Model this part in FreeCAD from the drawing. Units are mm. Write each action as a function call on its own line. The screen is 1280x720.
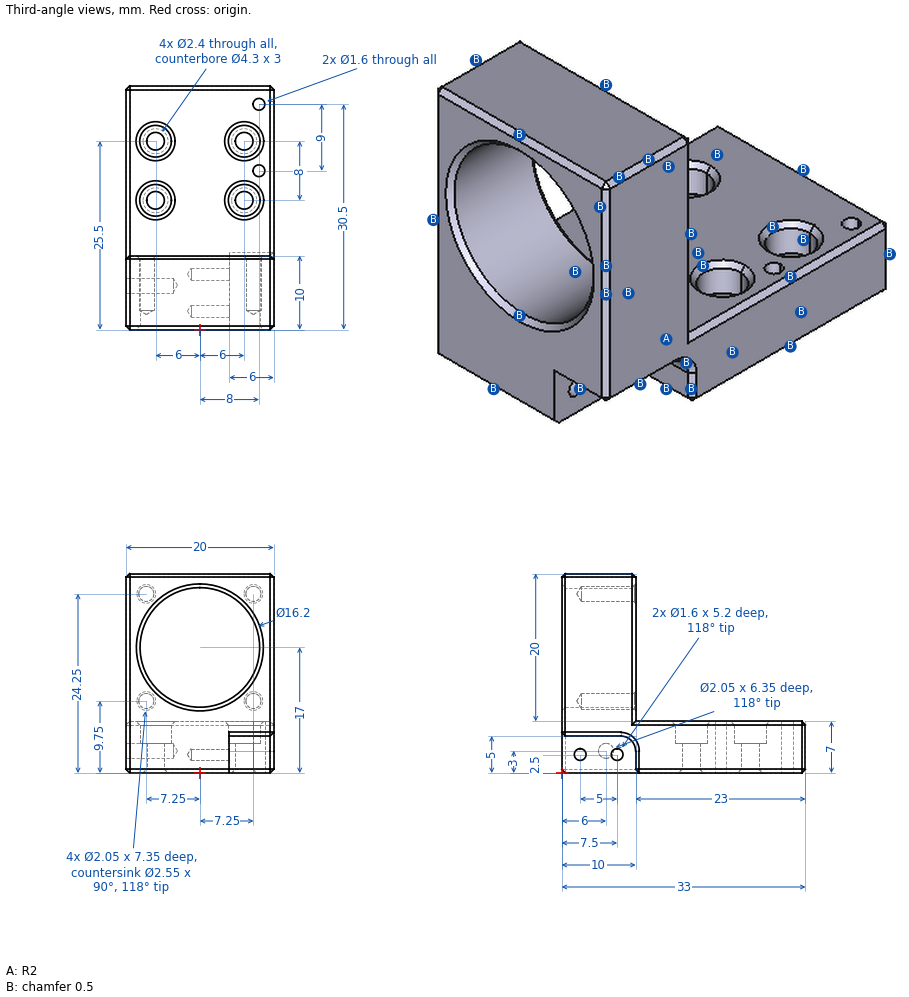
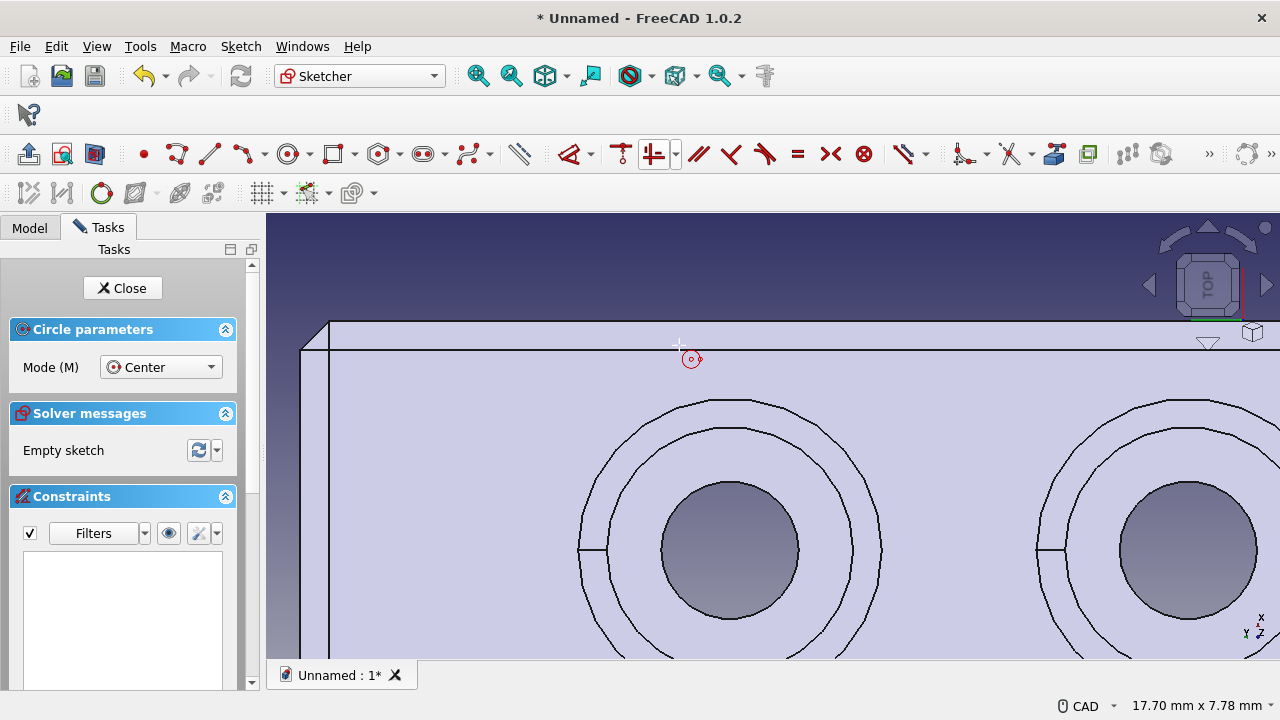
click(444, 436)
move(476, 403)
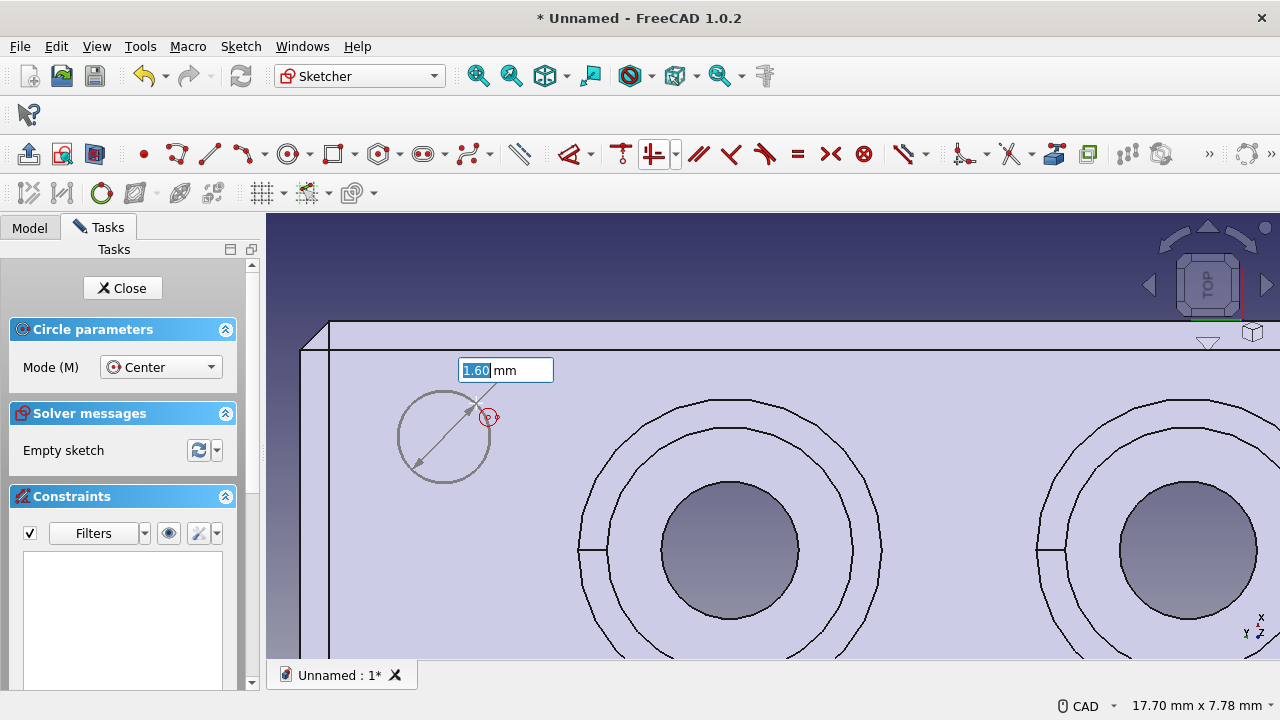
text(1.6)
key(Return)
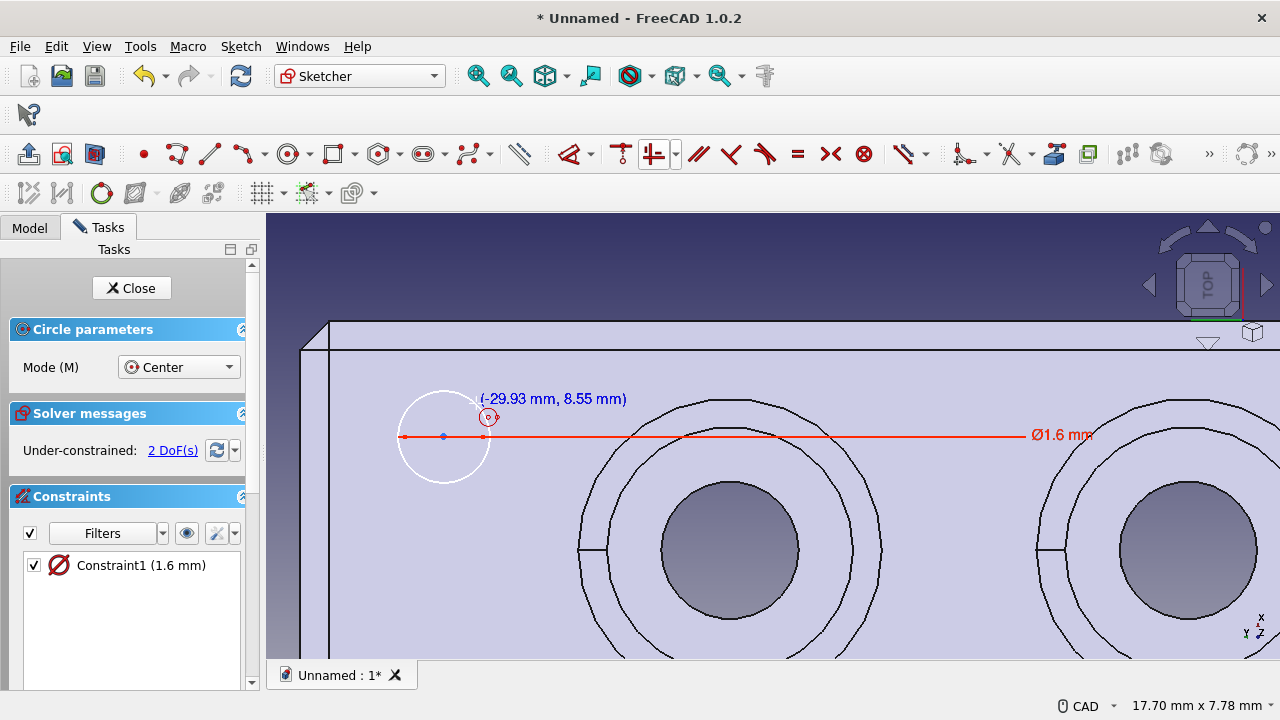
click(959, 436)
move(992, 403)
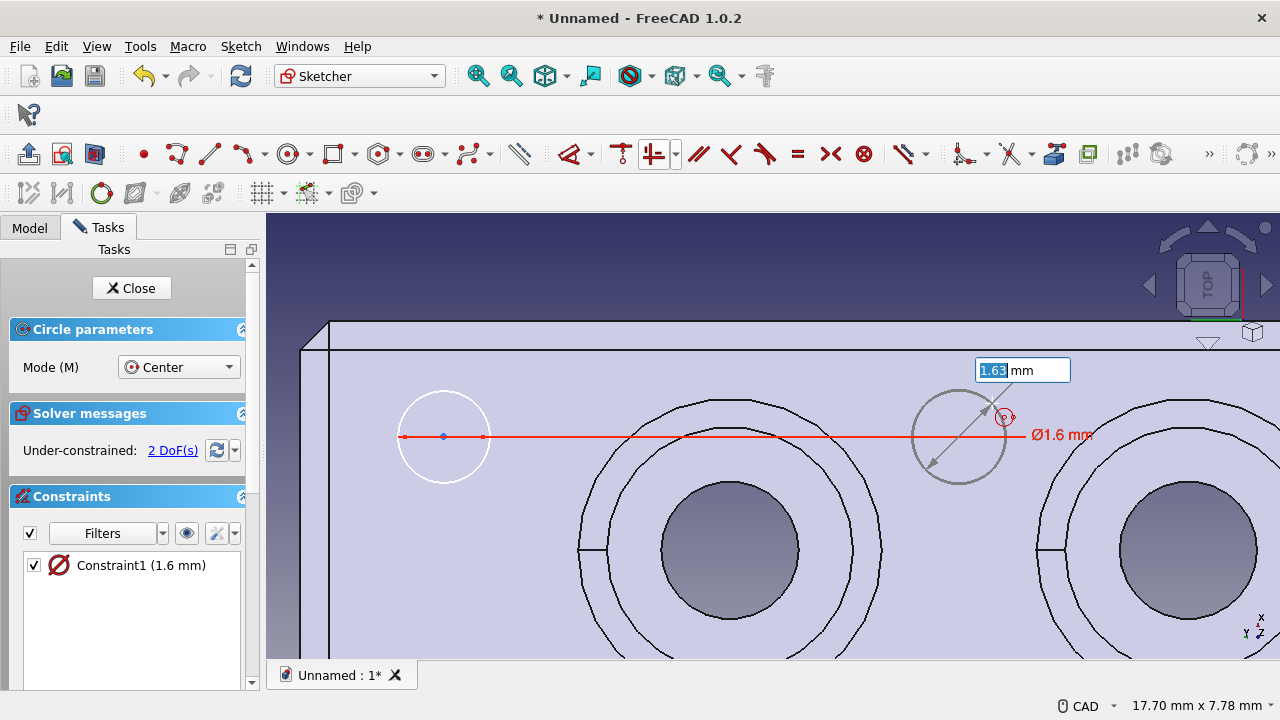
text(1.6)
key(Return)
key(Escape)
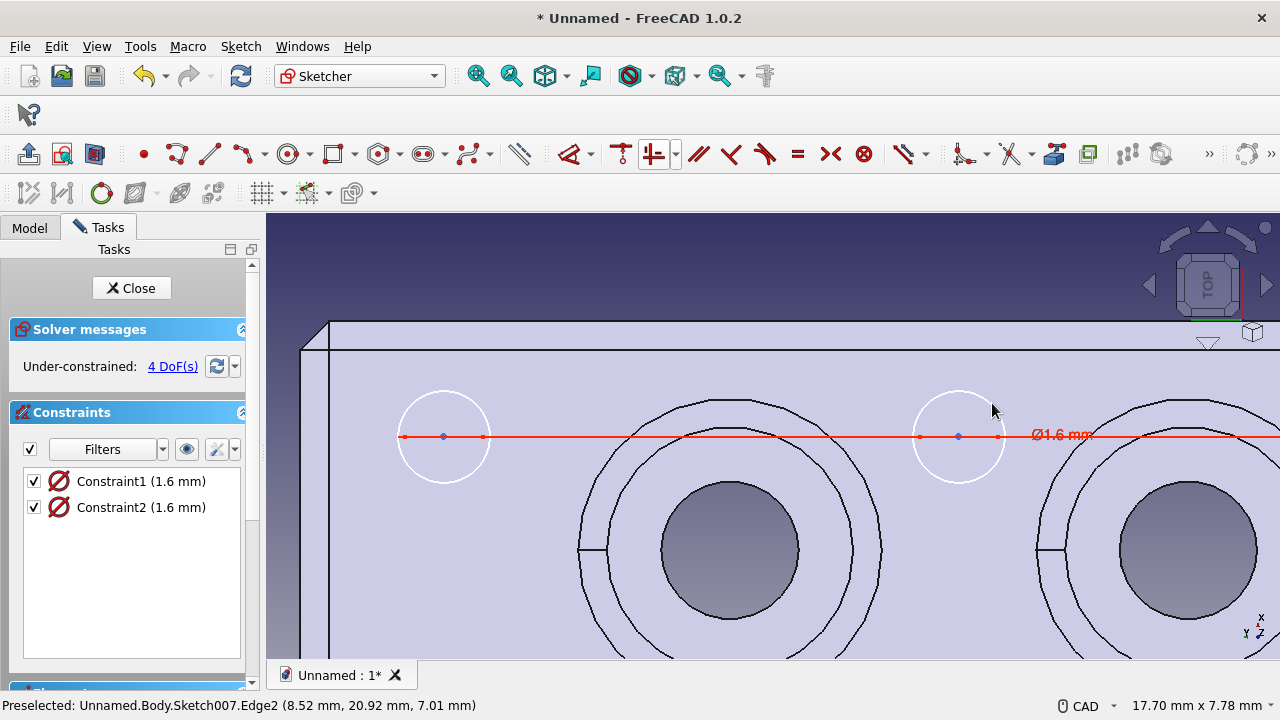
click(444, 437)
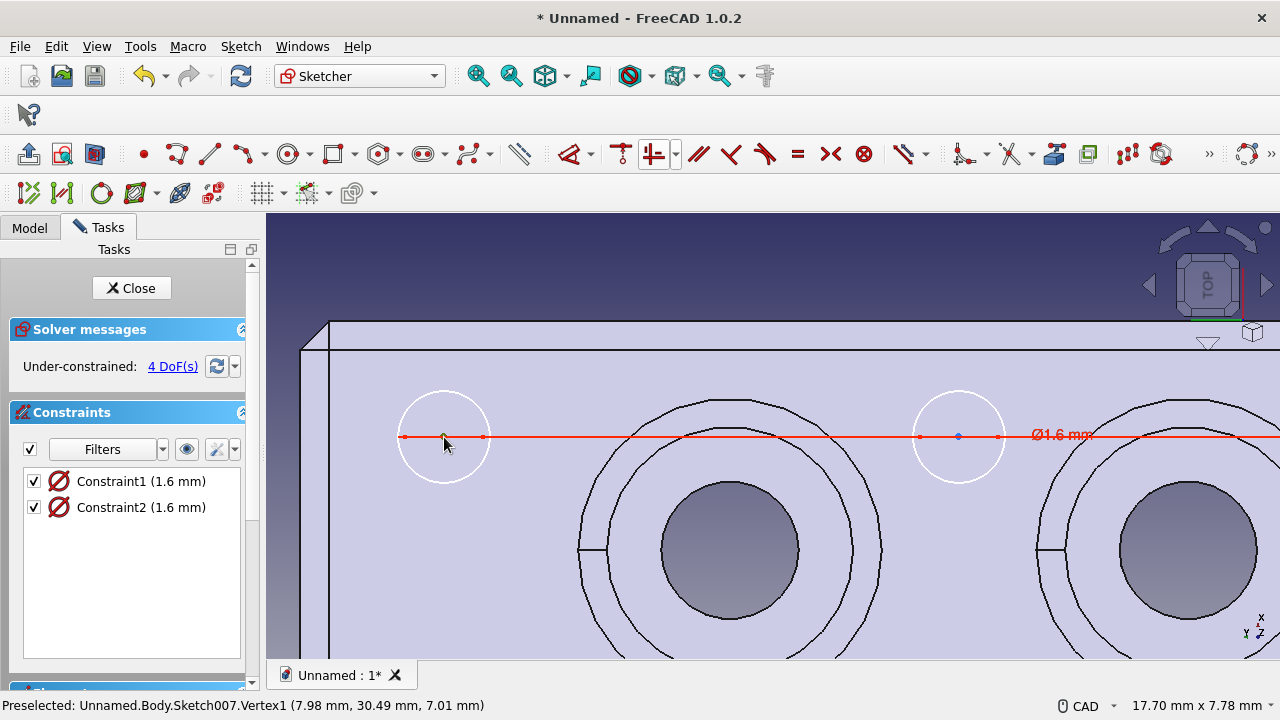
click(959, 437)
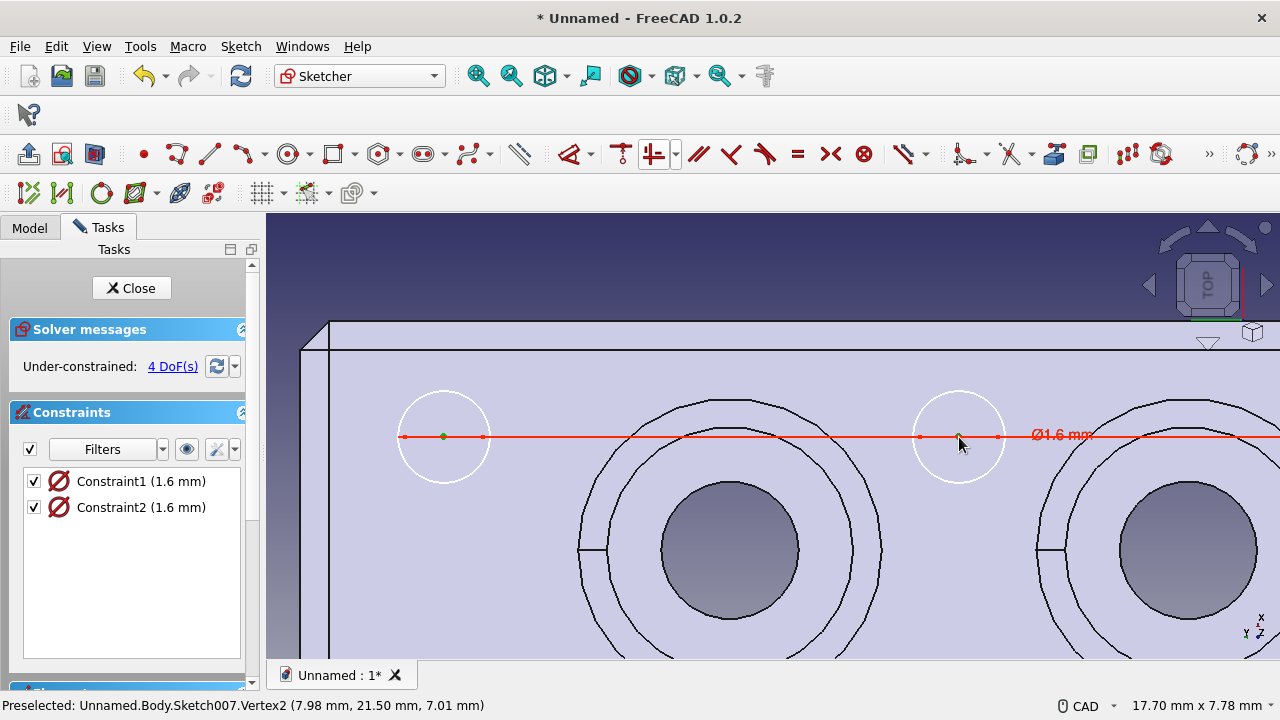
click(676, 154)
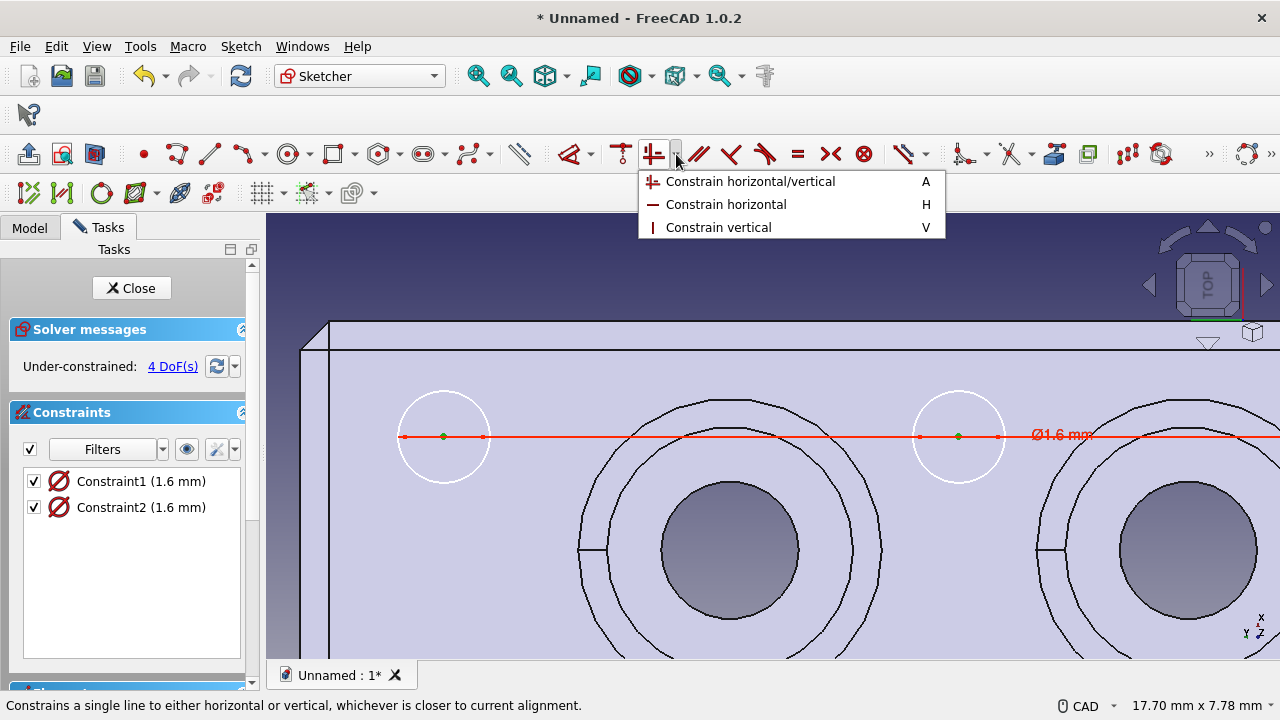
click(792, 204)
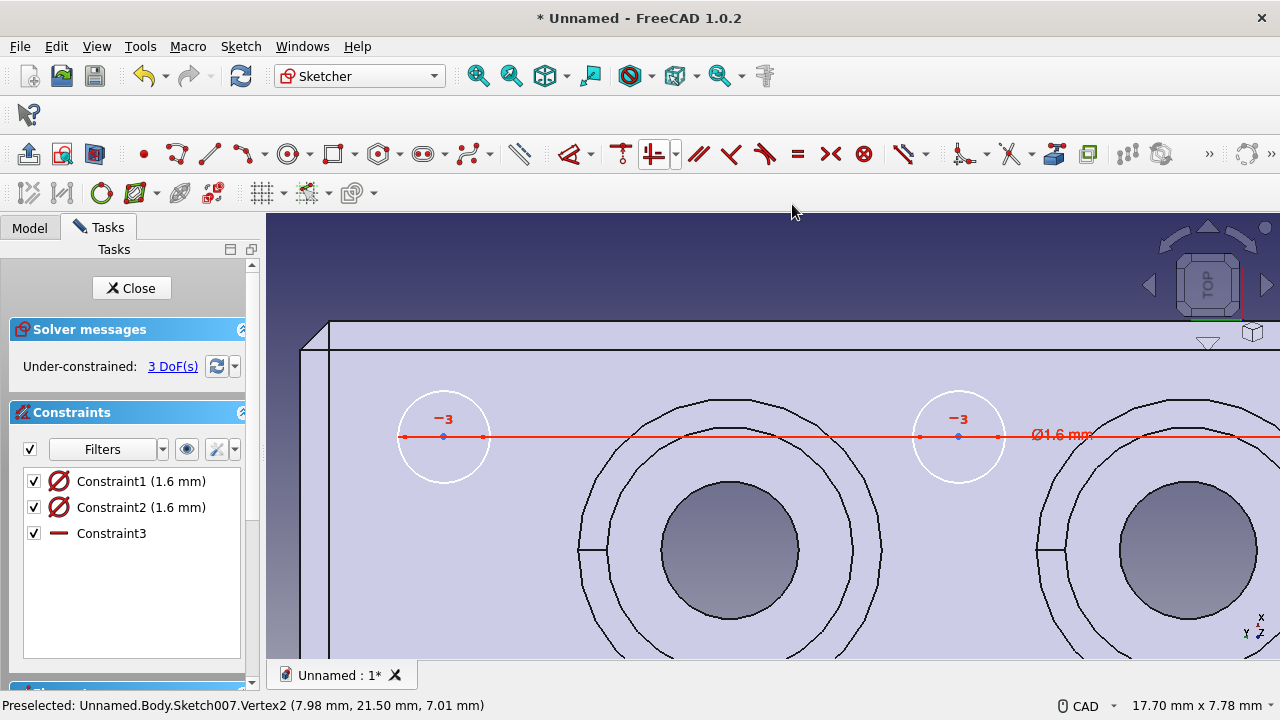
key(d)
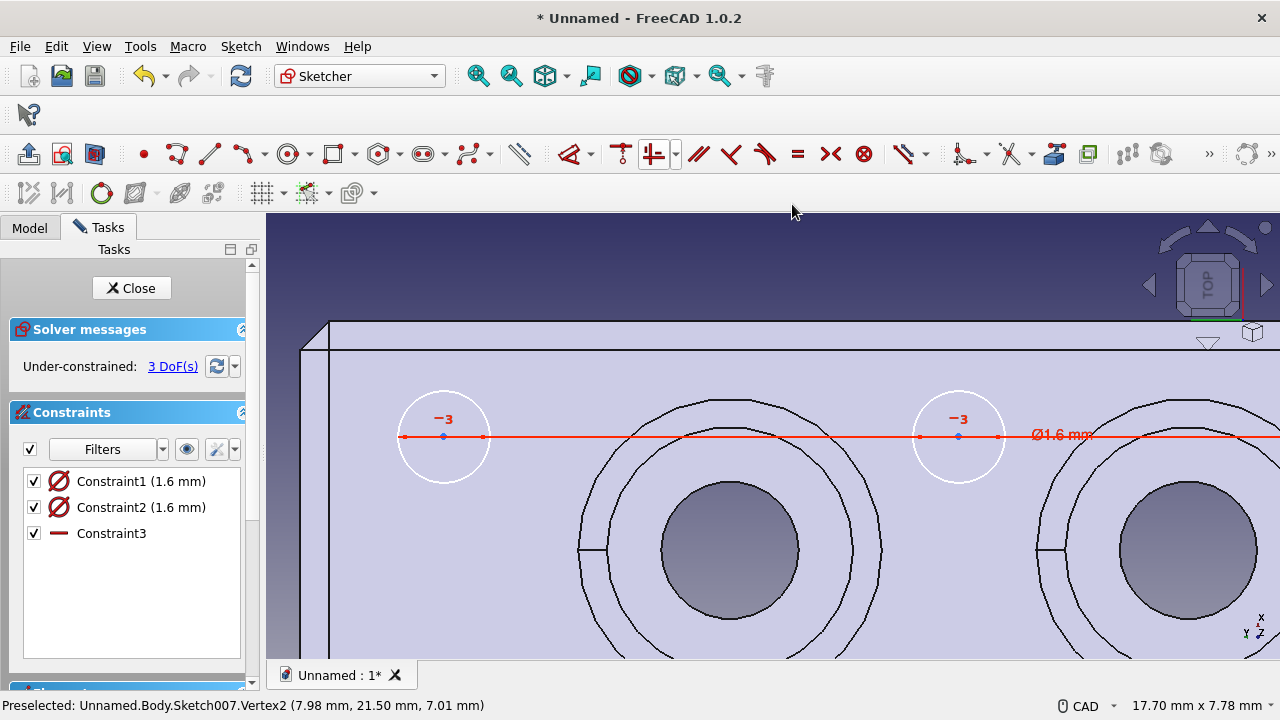
click(444, 437)
click(410, 534)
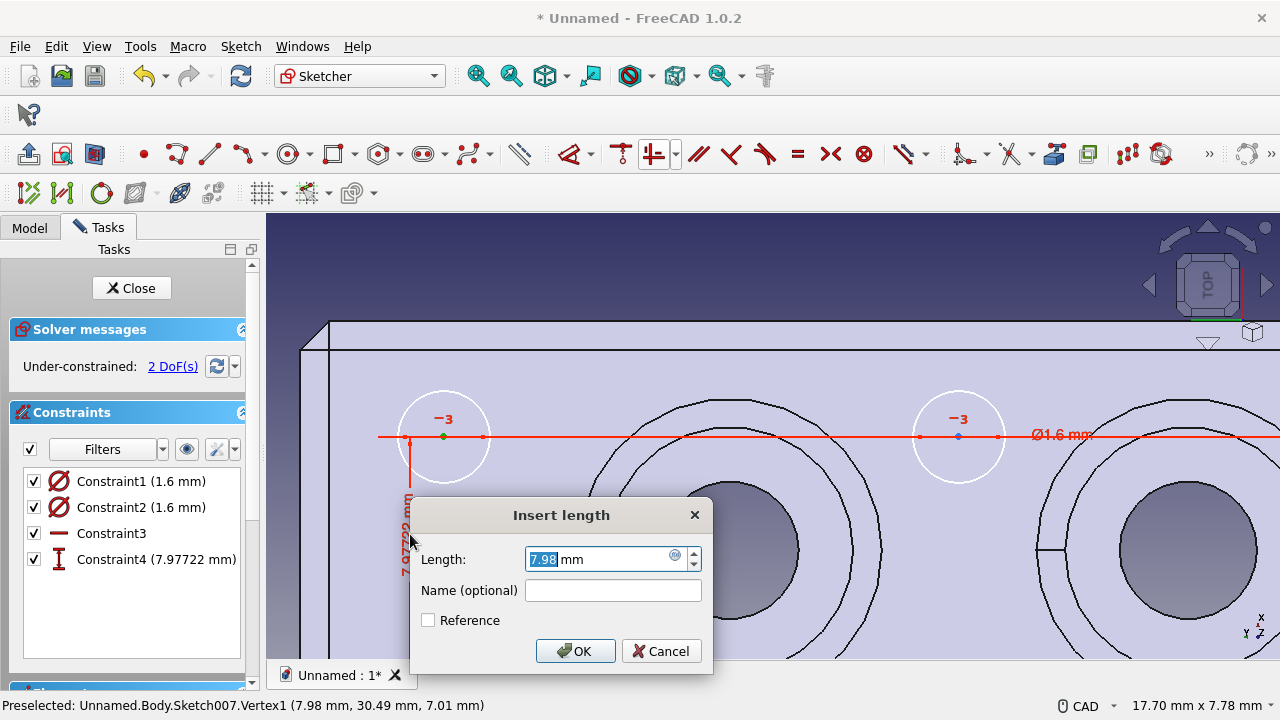
text(8)
key(Return)